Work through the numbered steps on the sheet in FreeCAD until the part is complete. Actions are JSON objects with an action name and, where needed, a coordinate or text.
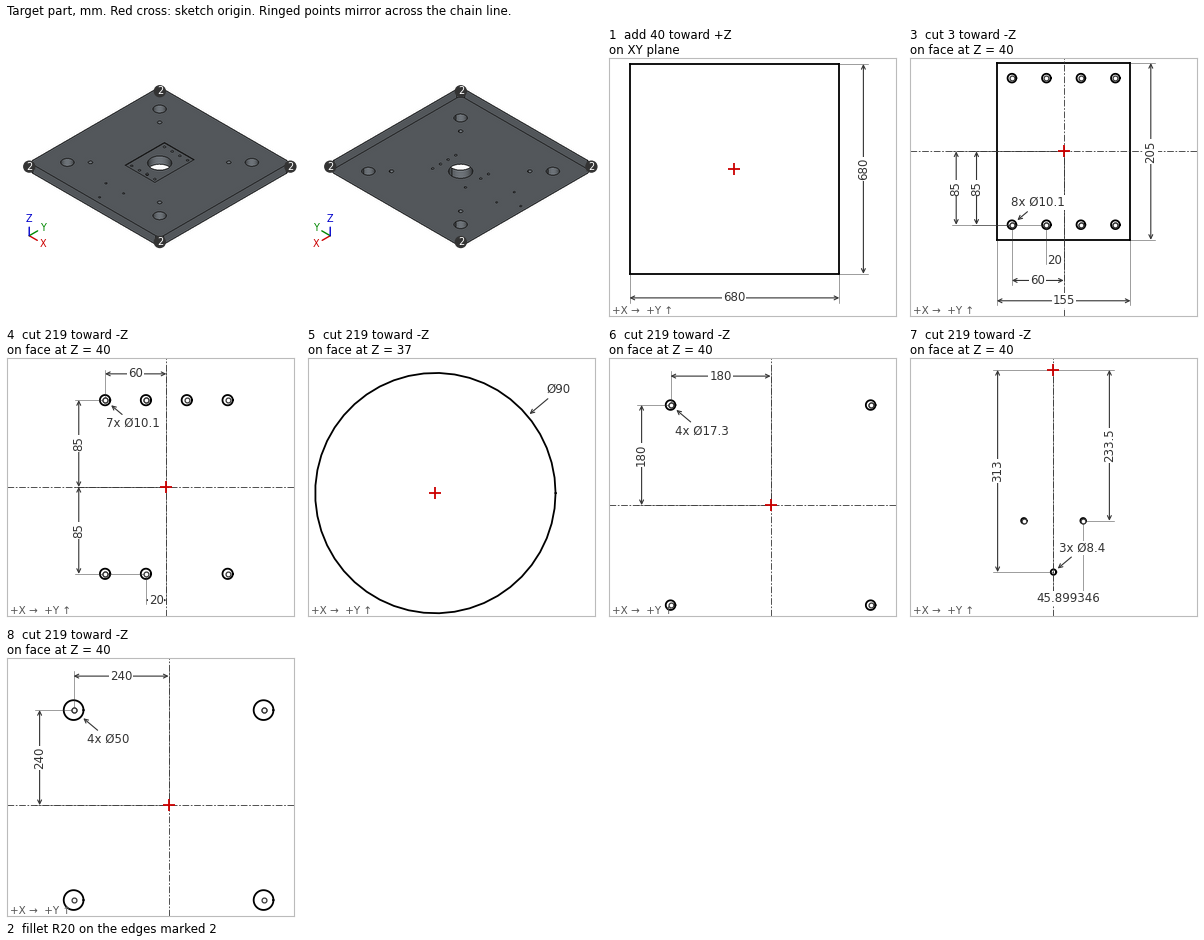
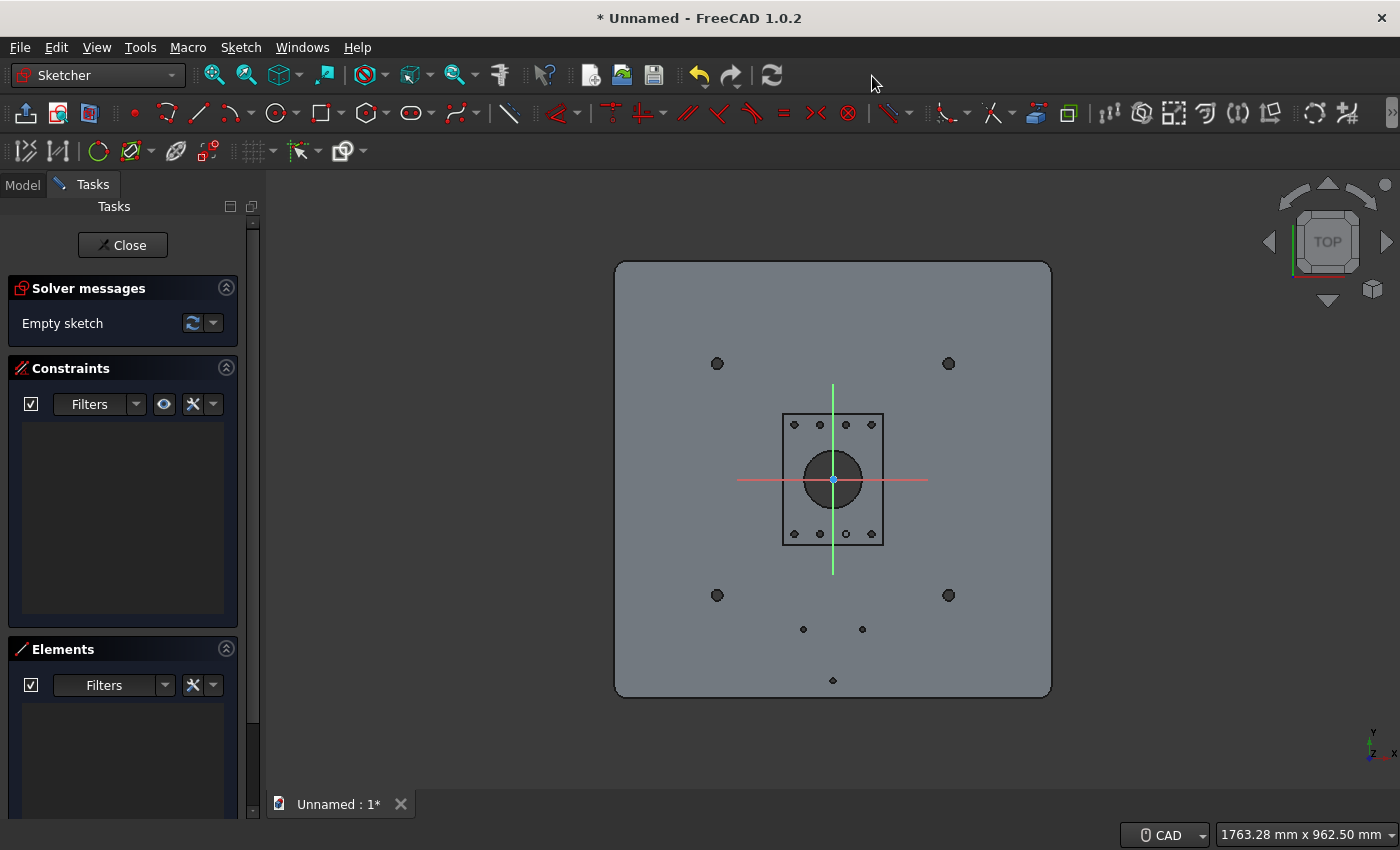
{"action": "left_click", "coordinate": [276, 114]}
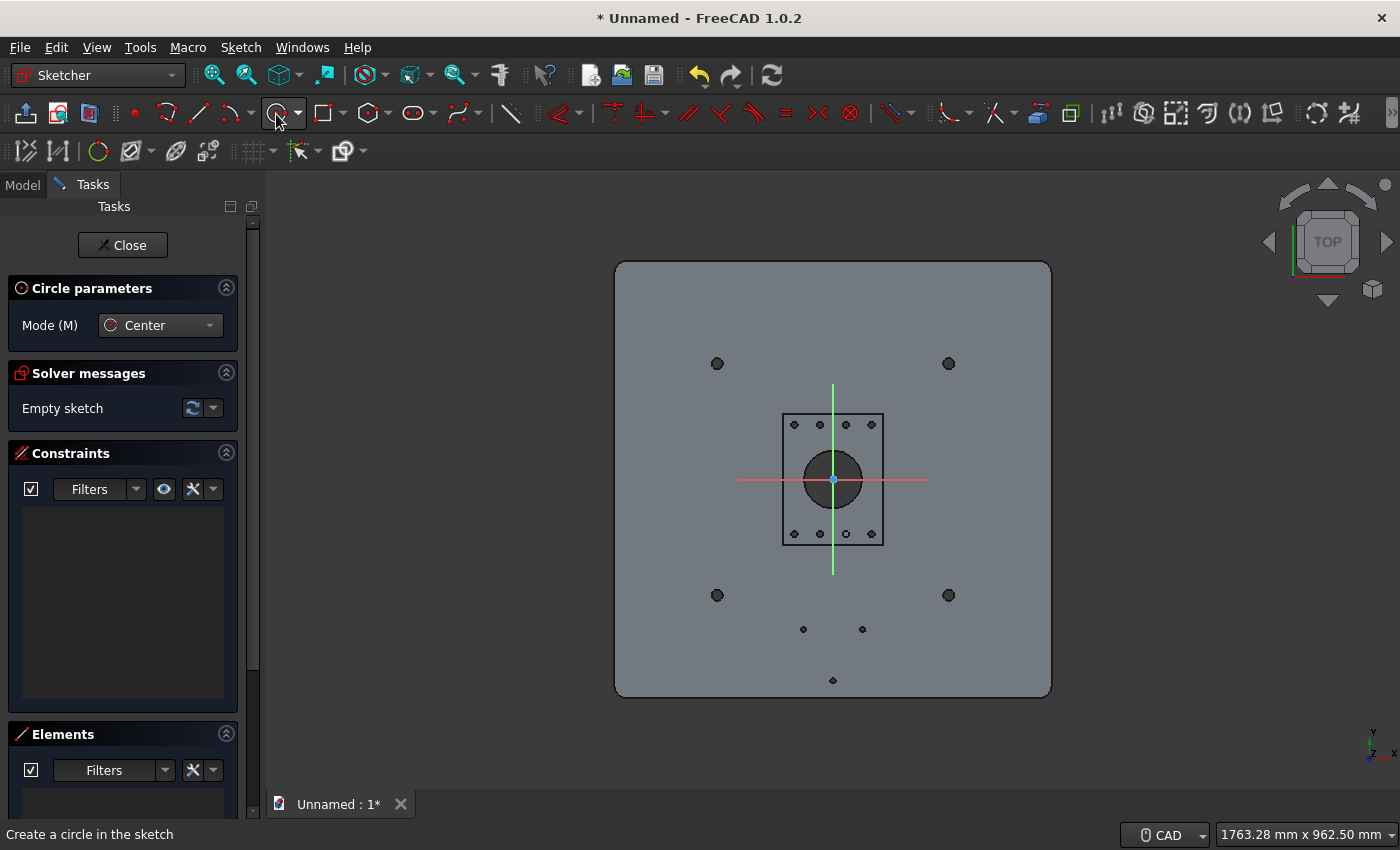
{"action": "scroll", "coordinate": [679, 325], "scroll_direction": "up", "scroll_amount": 2}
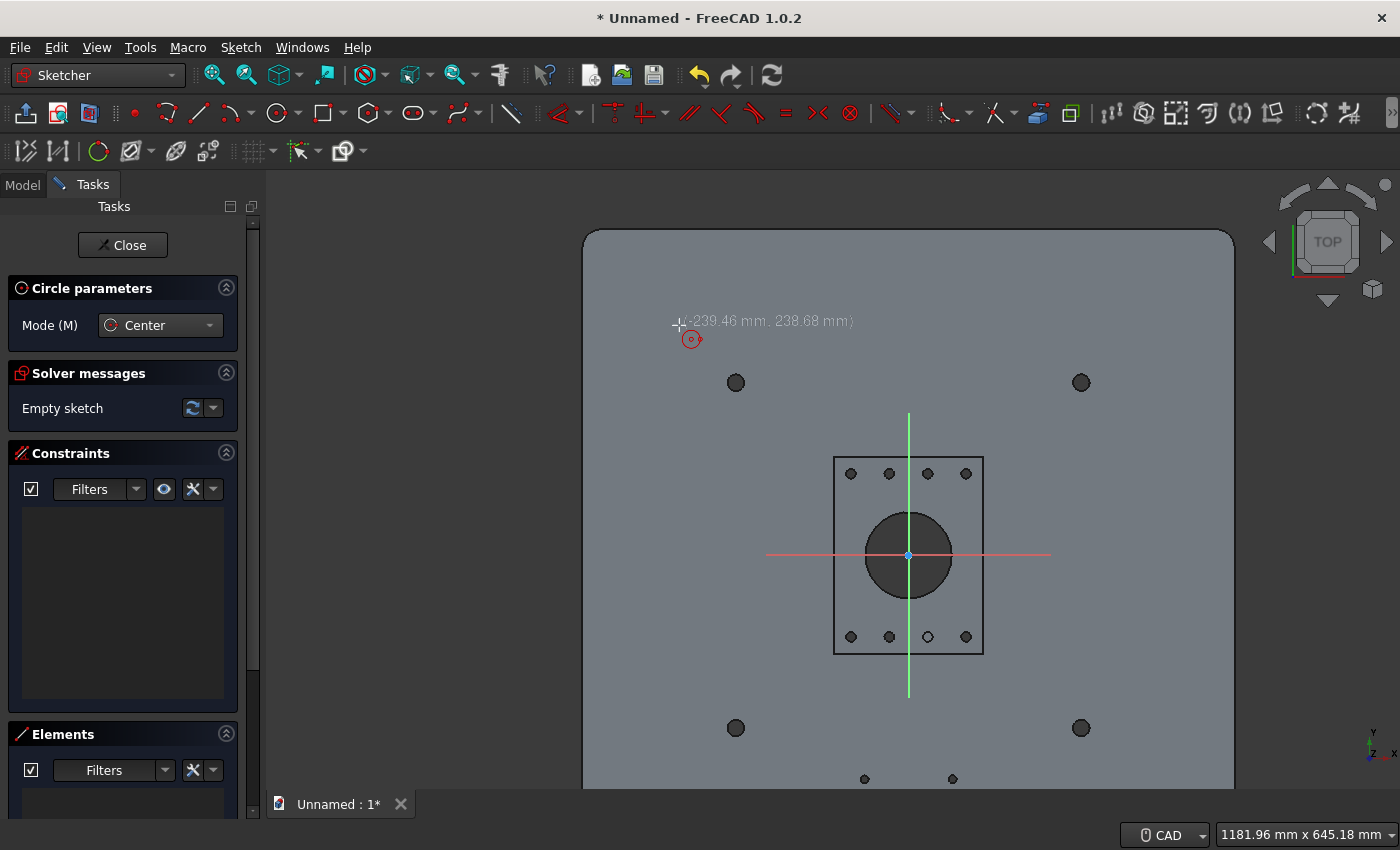
{"action": "left_click", "coordinate": [678, 325]}
{"action": "left_click", "coordinate": [695, 308]}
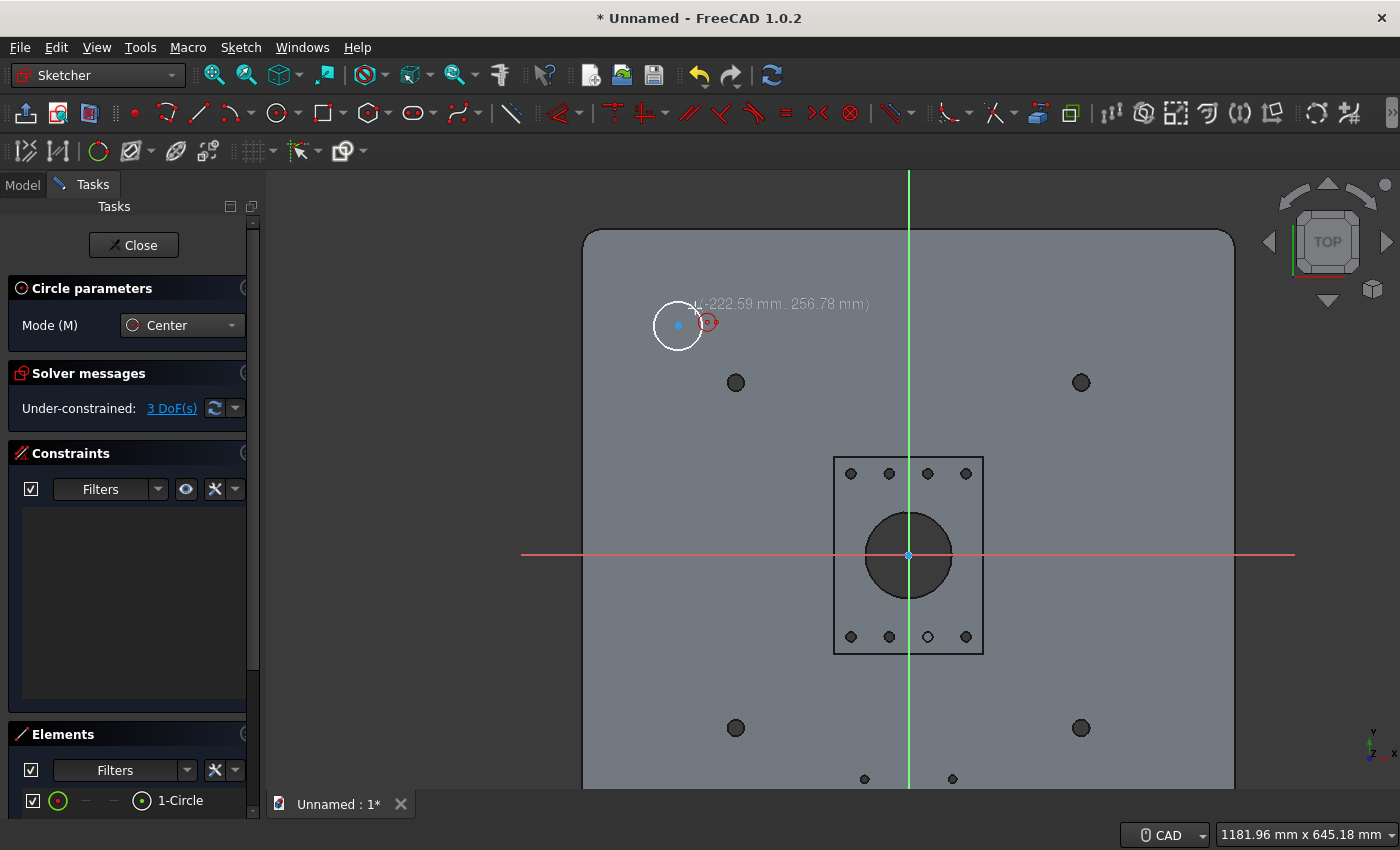
{"action": "left_click", "coordinate": [1139, 325]}
{"action": "left_click", "coordinate": [1156, 308]}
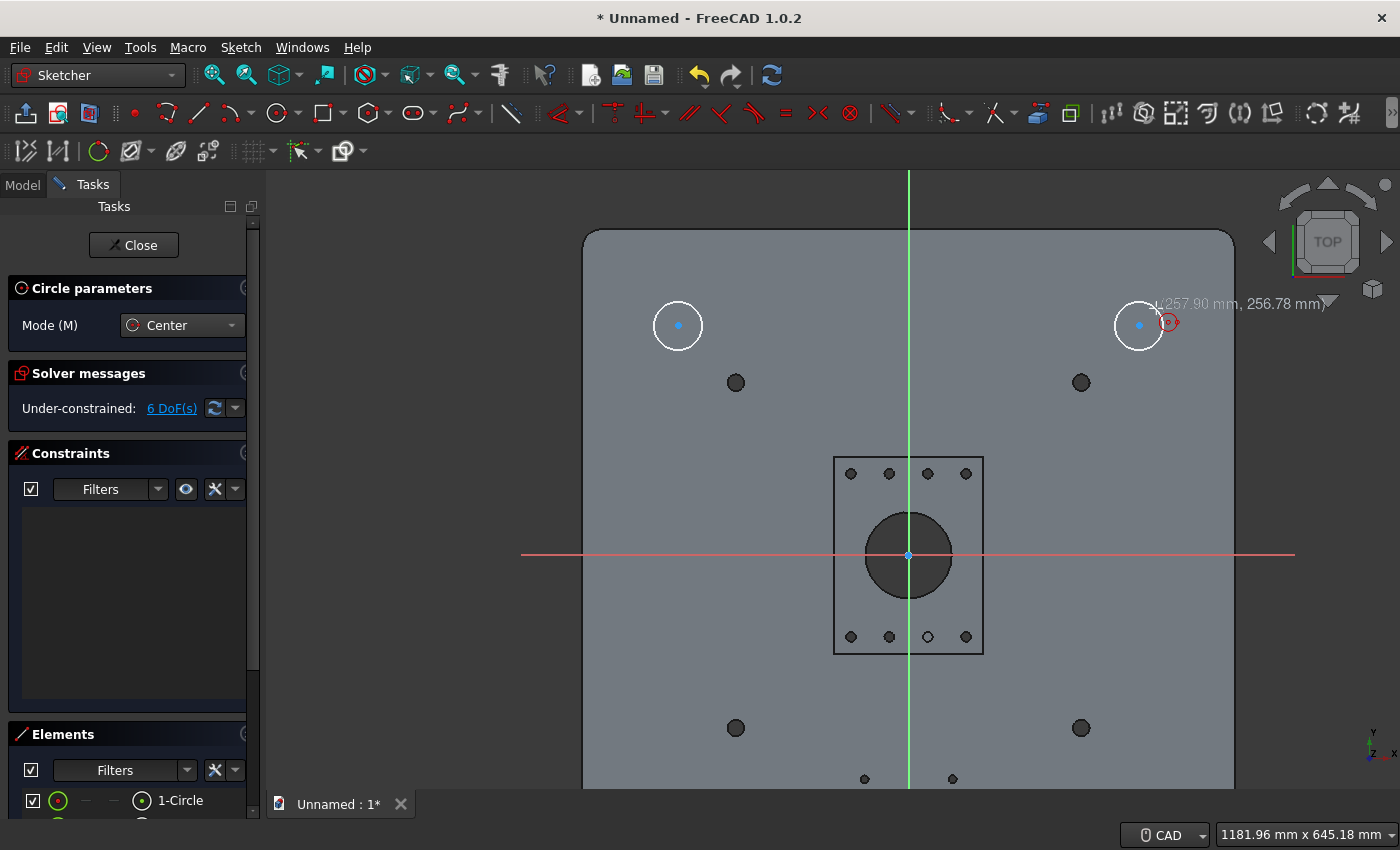
{"action": "scroll", "coordinate": [294, 198], "scroll_direction": "down", "scroll_amount": 1}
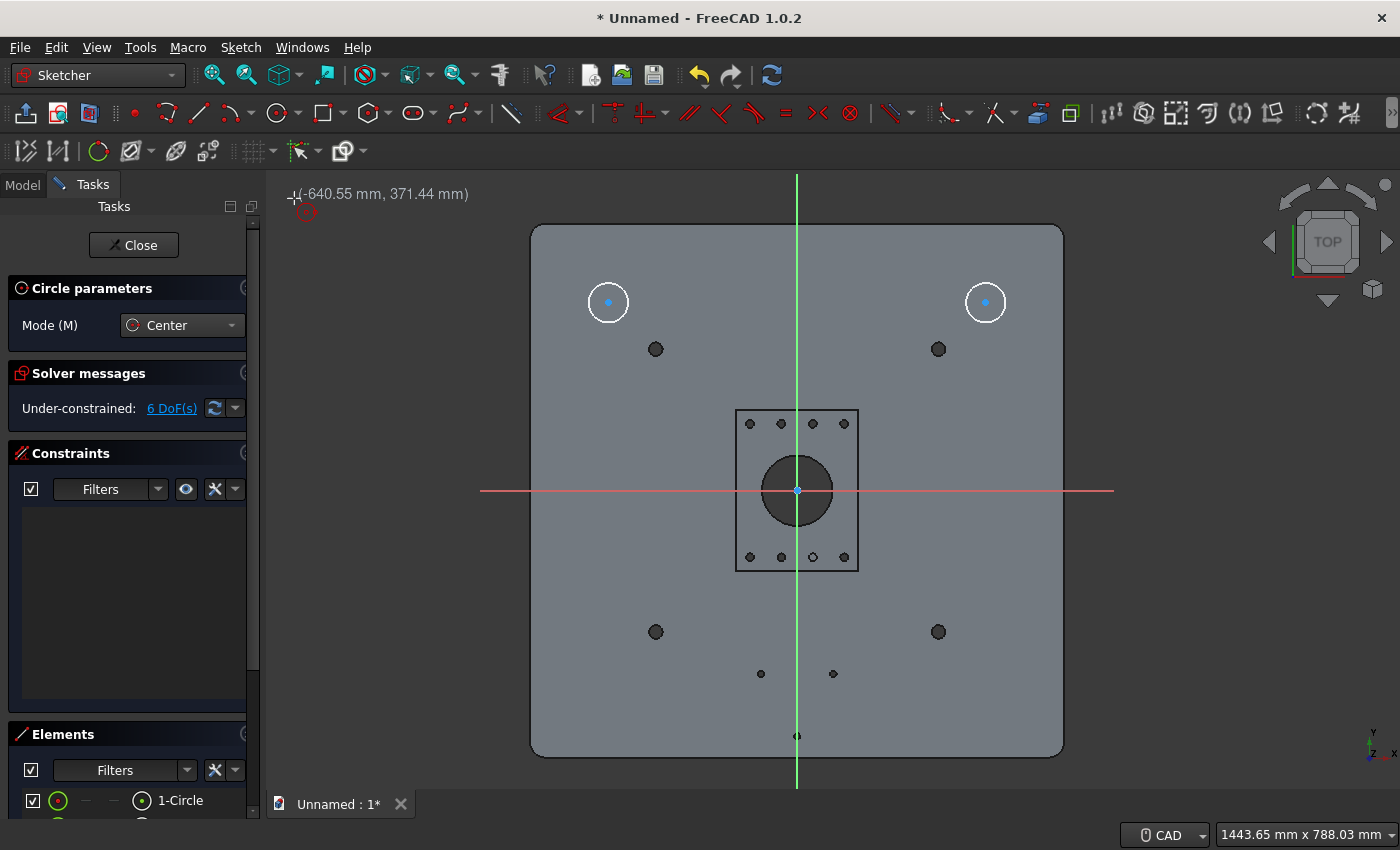
{"action": "left_click", "coordinate": [986, 679]}
{"action": "left_click", "coordinate": [1000, 665]}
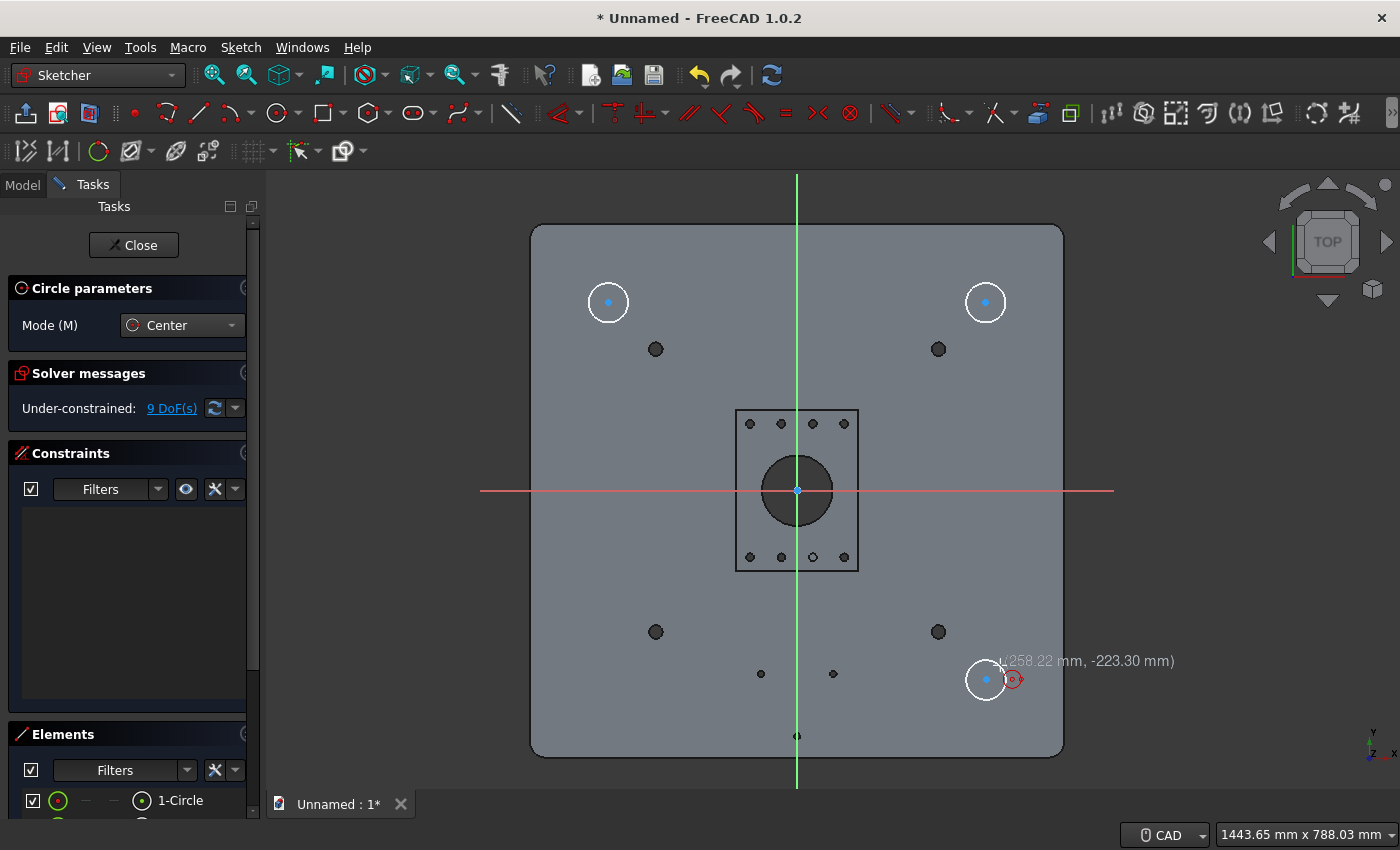
{"action": "left_click", "coordinate": [609, 679]}
{"action": "left_click", "coordinate": [623, 665]}
{"action": "key", "text": "Escape"}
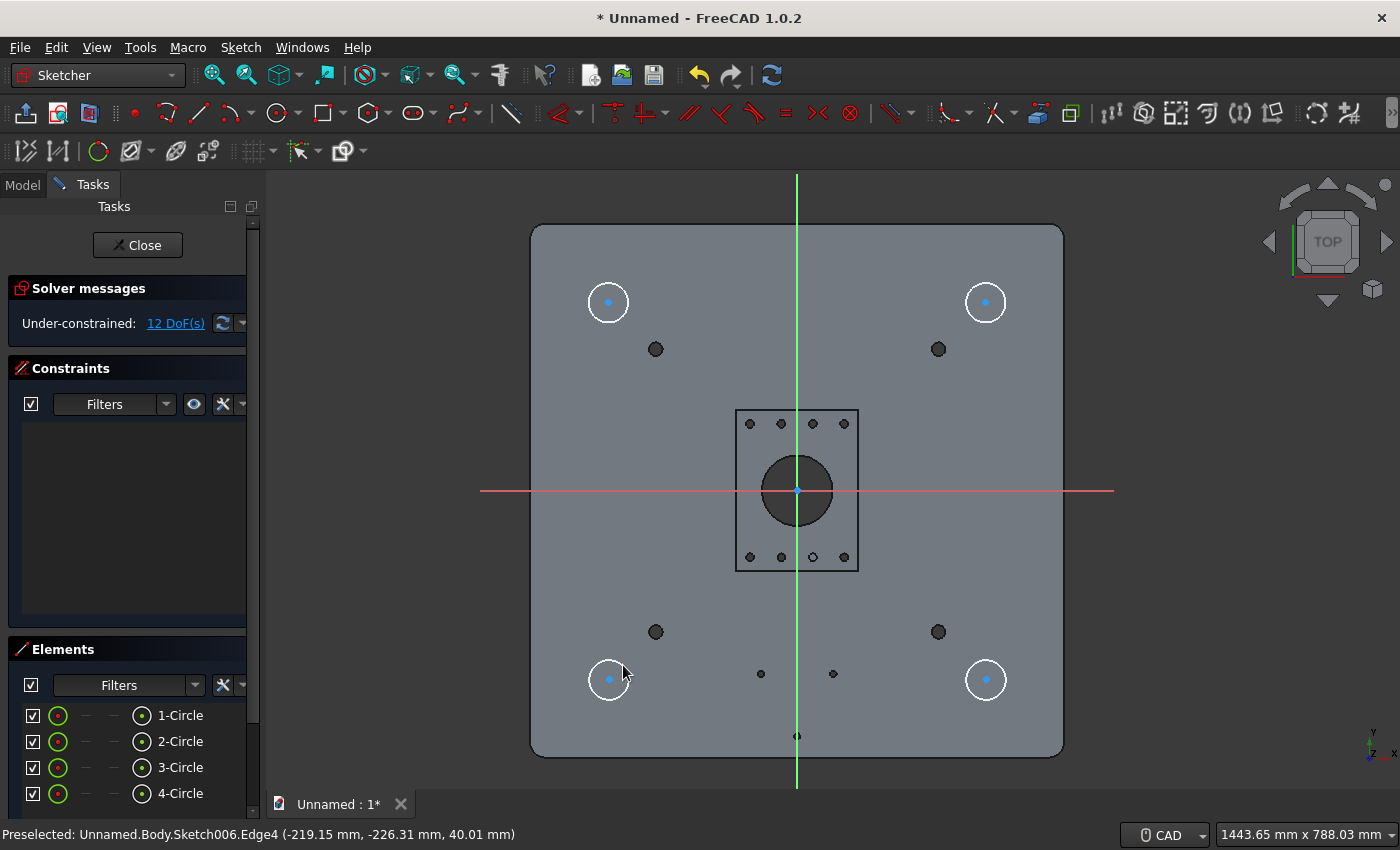
{"action": "left_click", "coordinate": [622, 289]}